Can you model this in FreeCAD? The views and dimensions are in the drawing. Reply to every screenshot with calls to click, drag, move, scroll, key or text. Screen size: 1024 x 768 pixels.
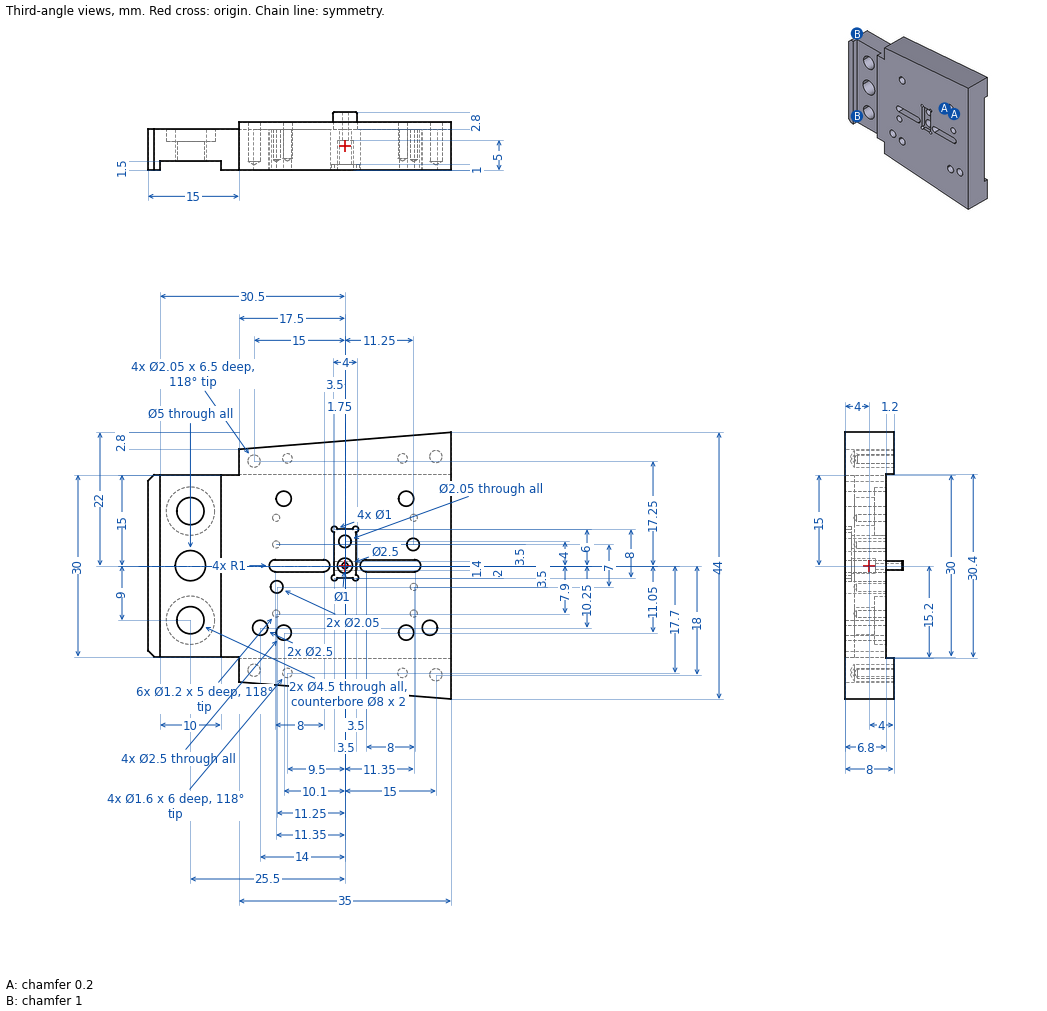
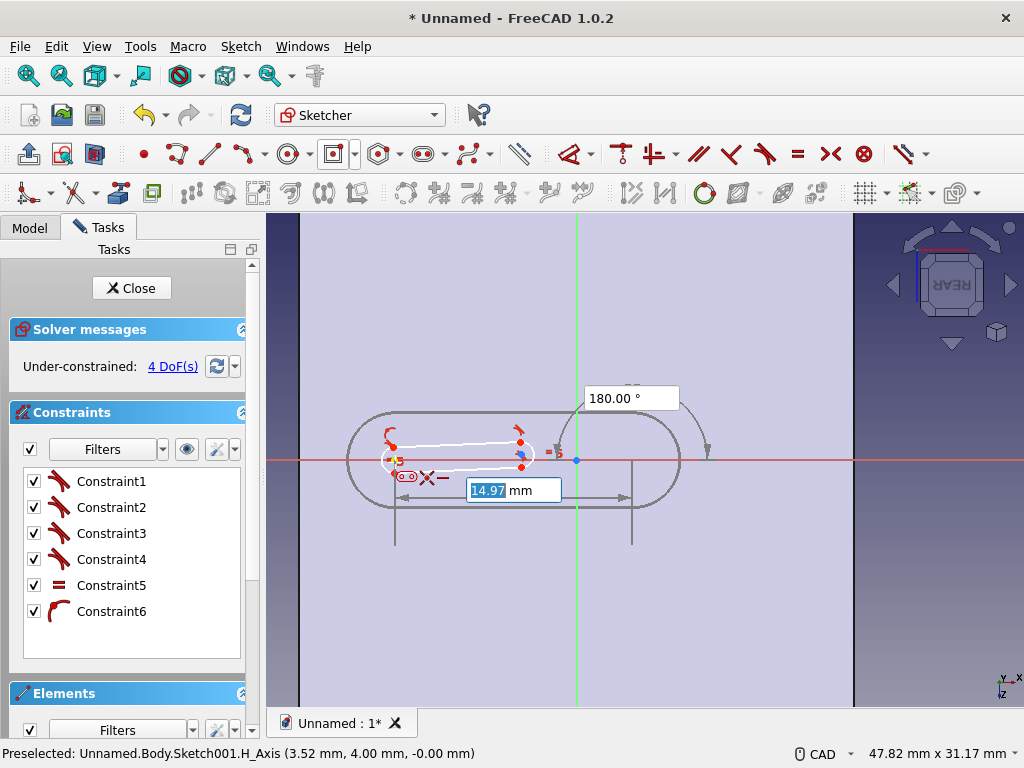
click(759, 451)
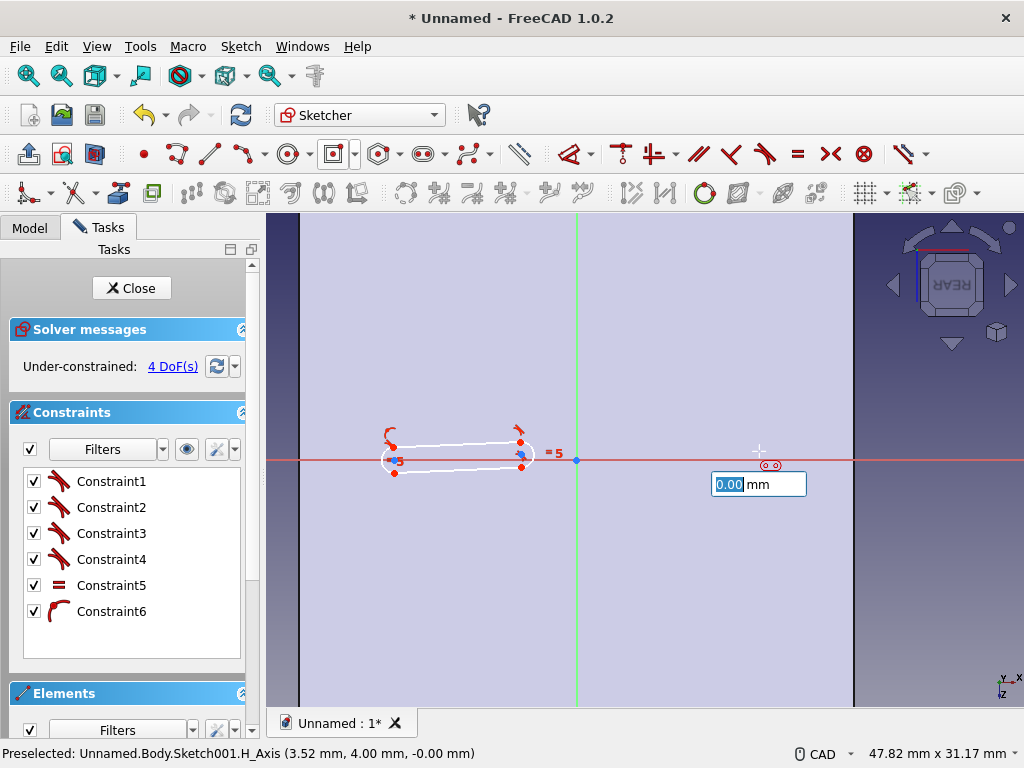
click(695, 444)
key(Escape)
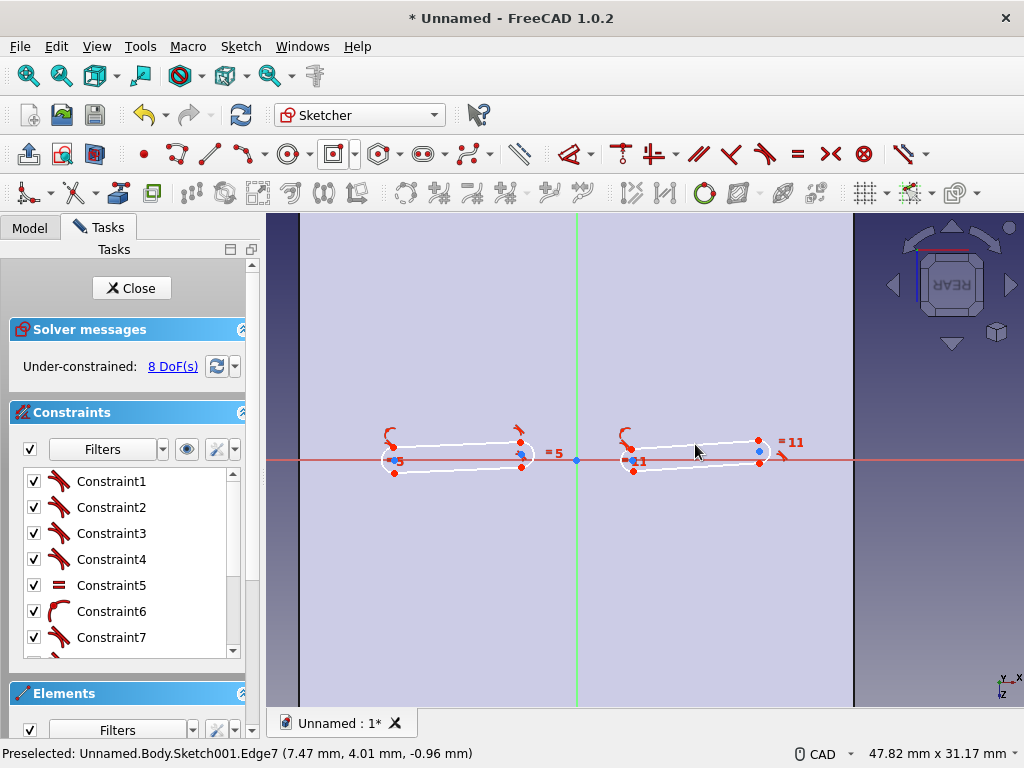
click(432, 446)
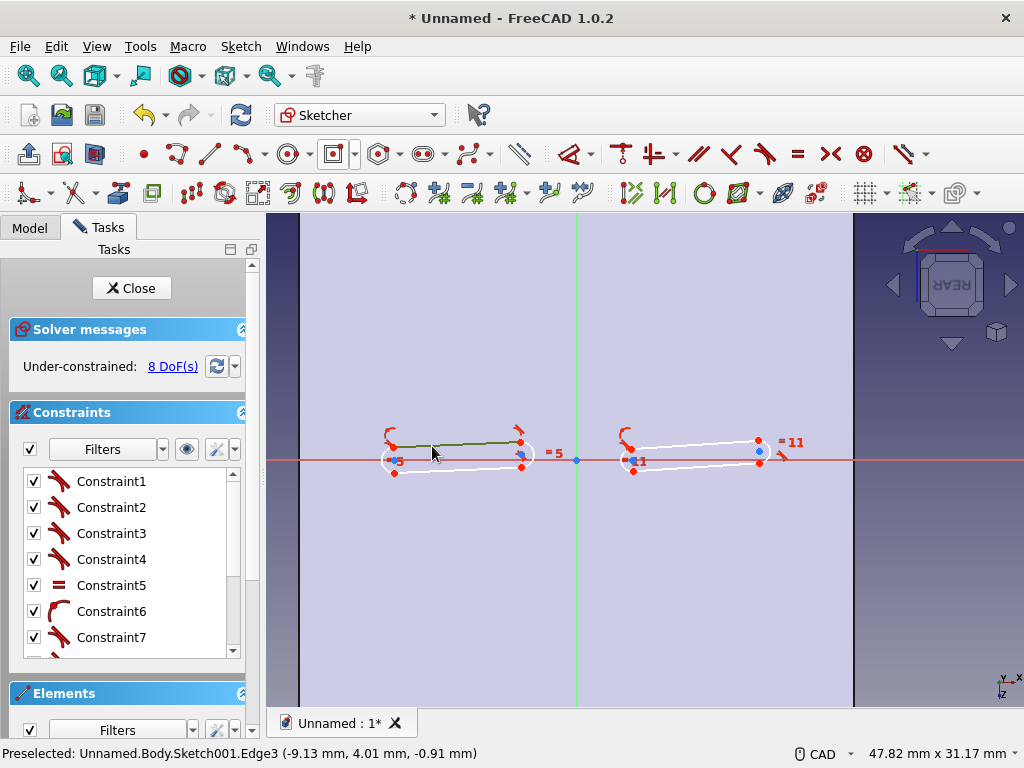
click(676, 154)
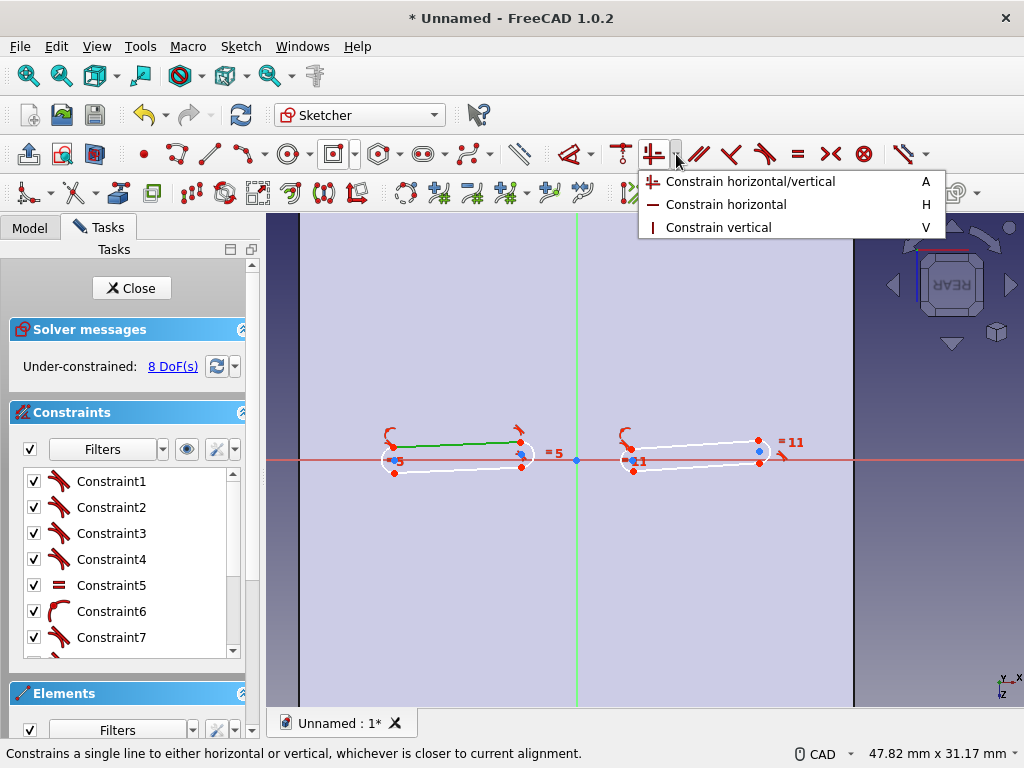
click(792, 204)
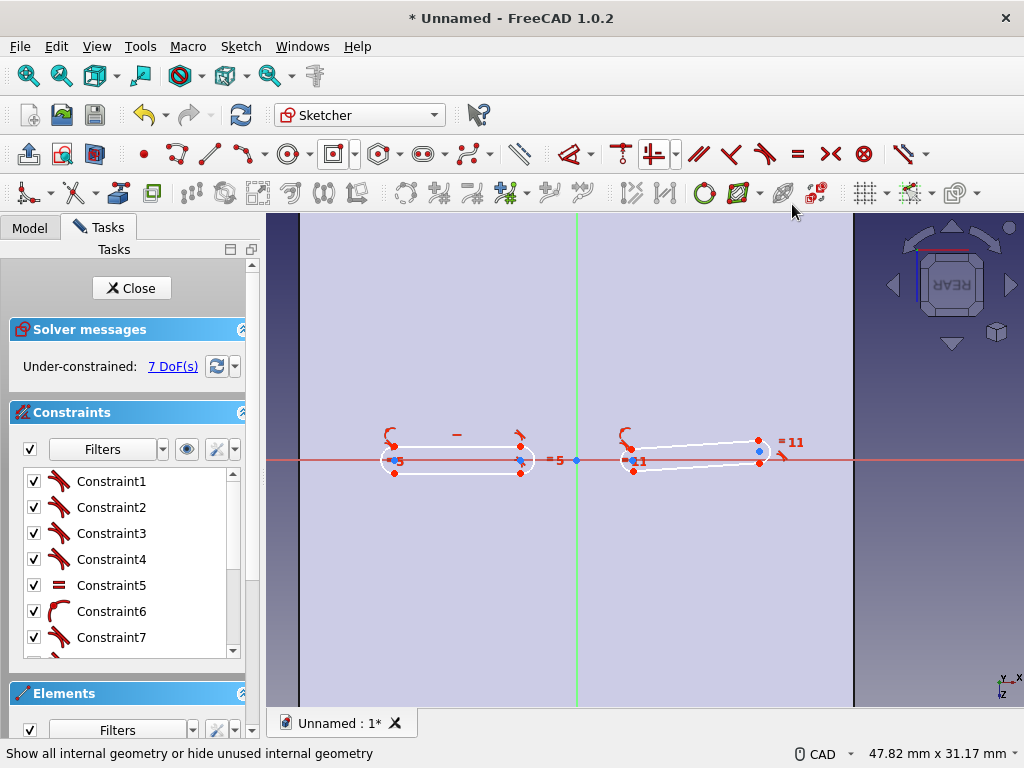
click(670, 447)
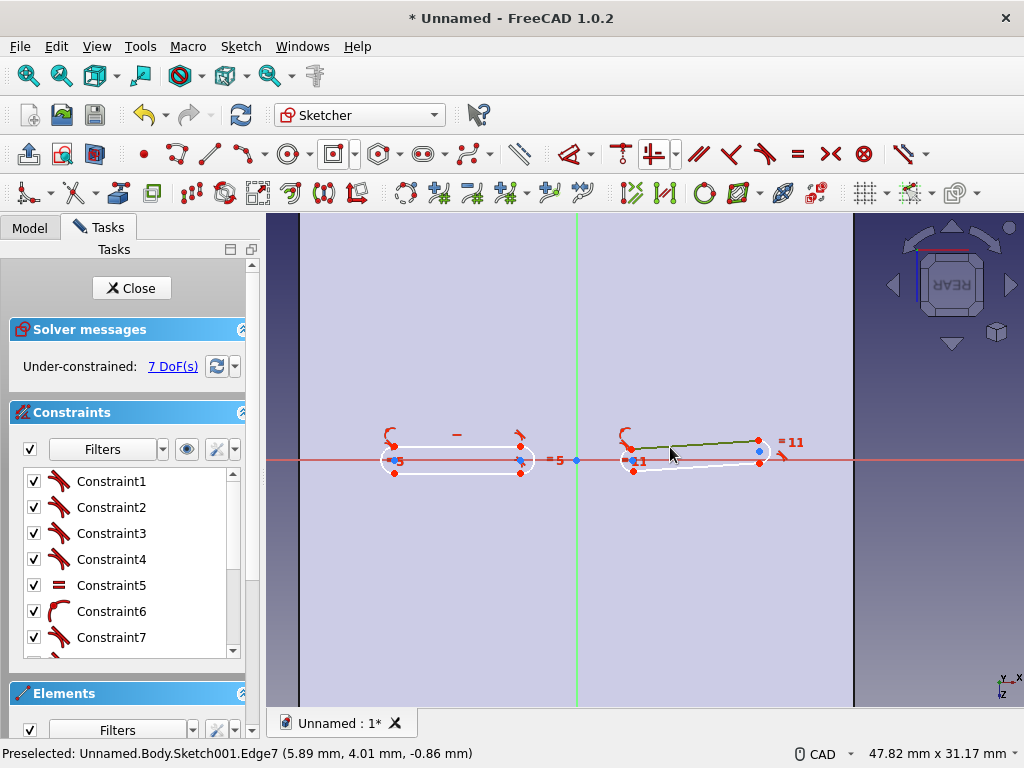
click(676, 154)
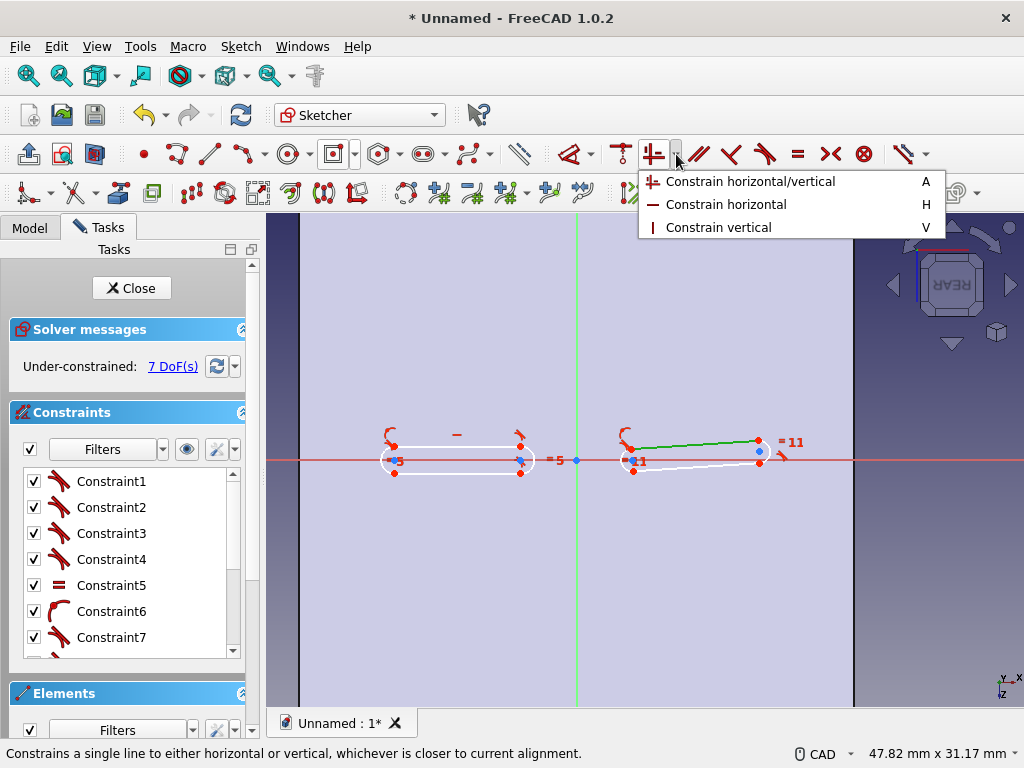
click(792, 204)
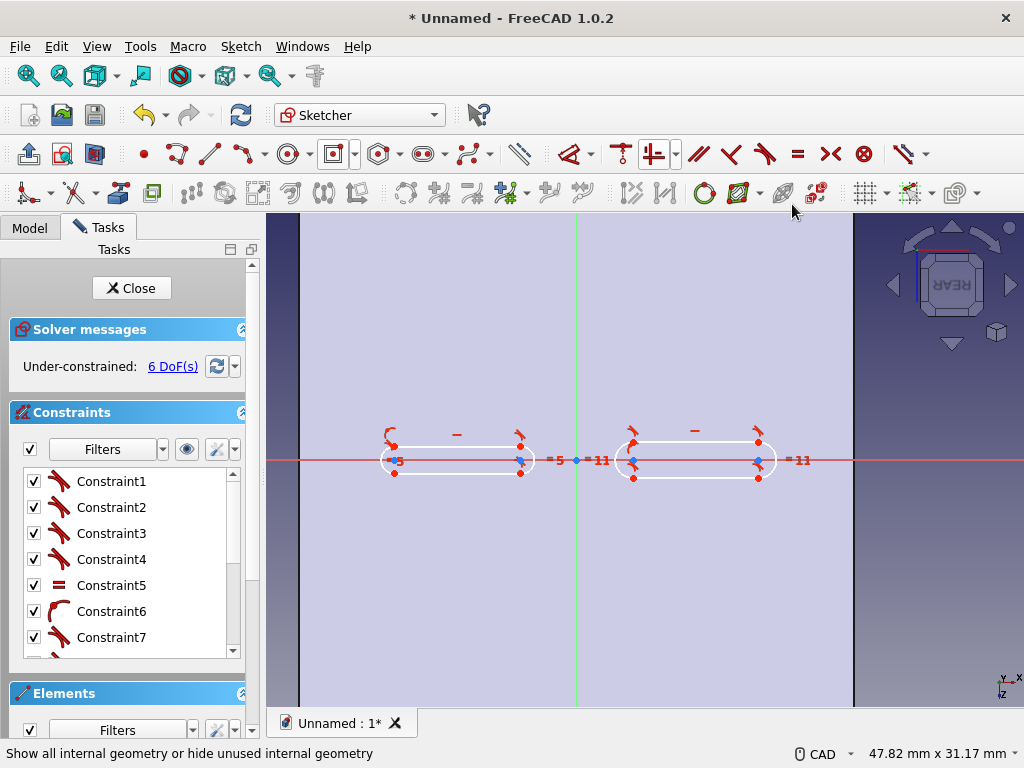
click(381, 460)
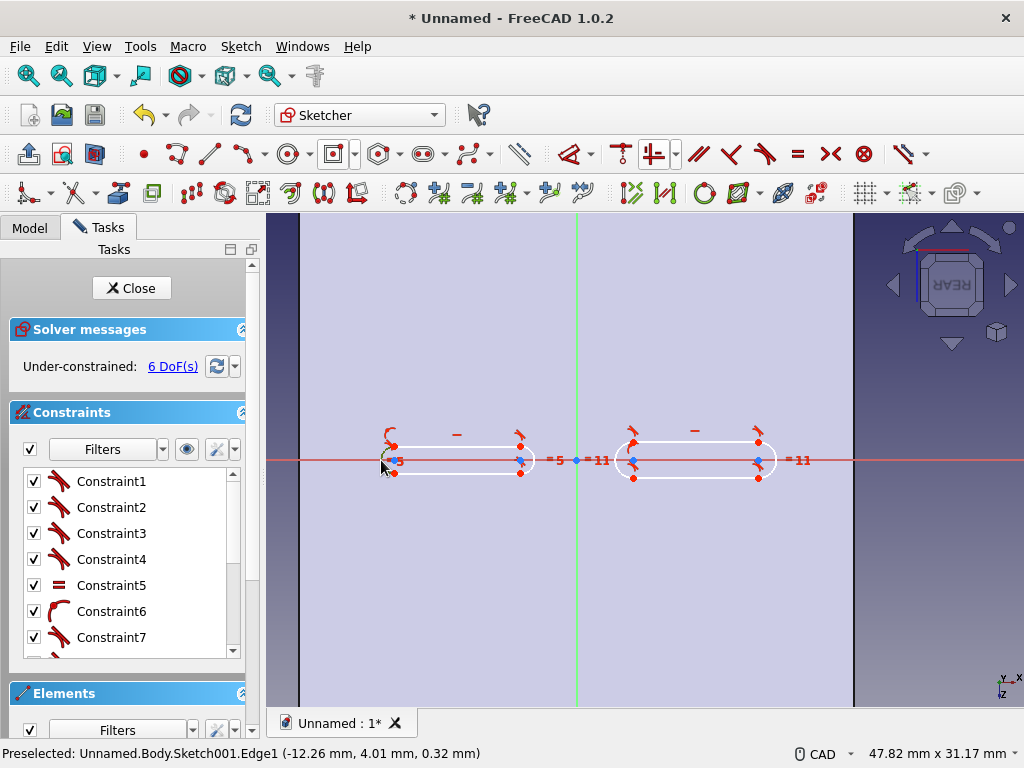
scroll(619, 450, up, 2)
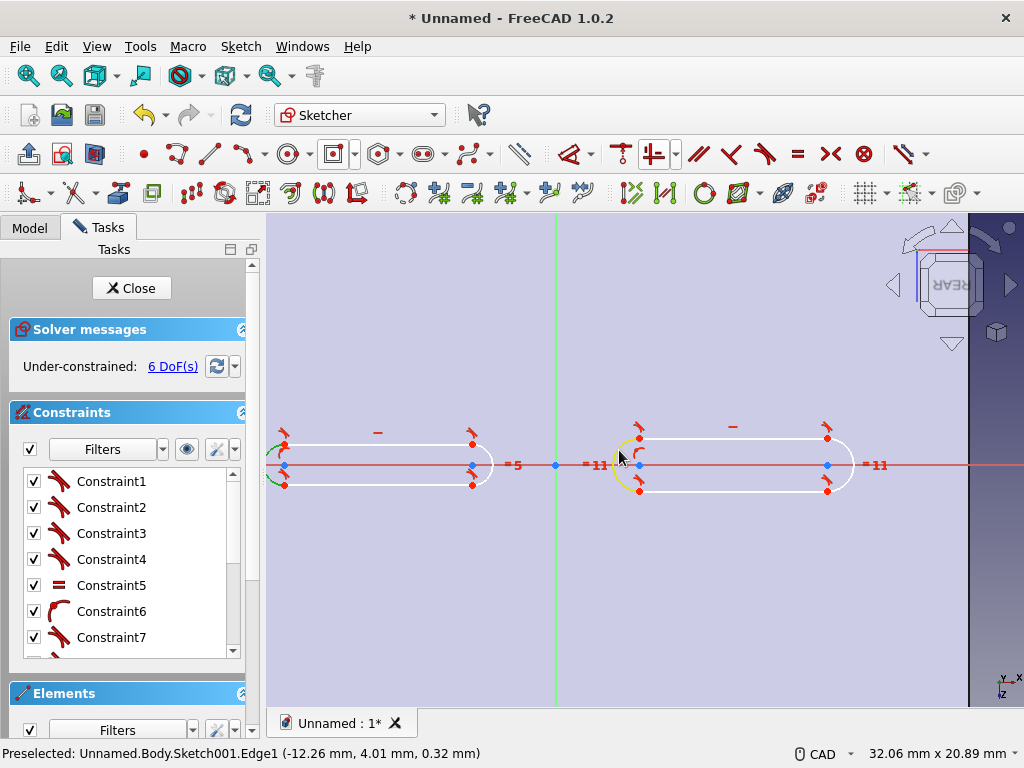
click(618, 449)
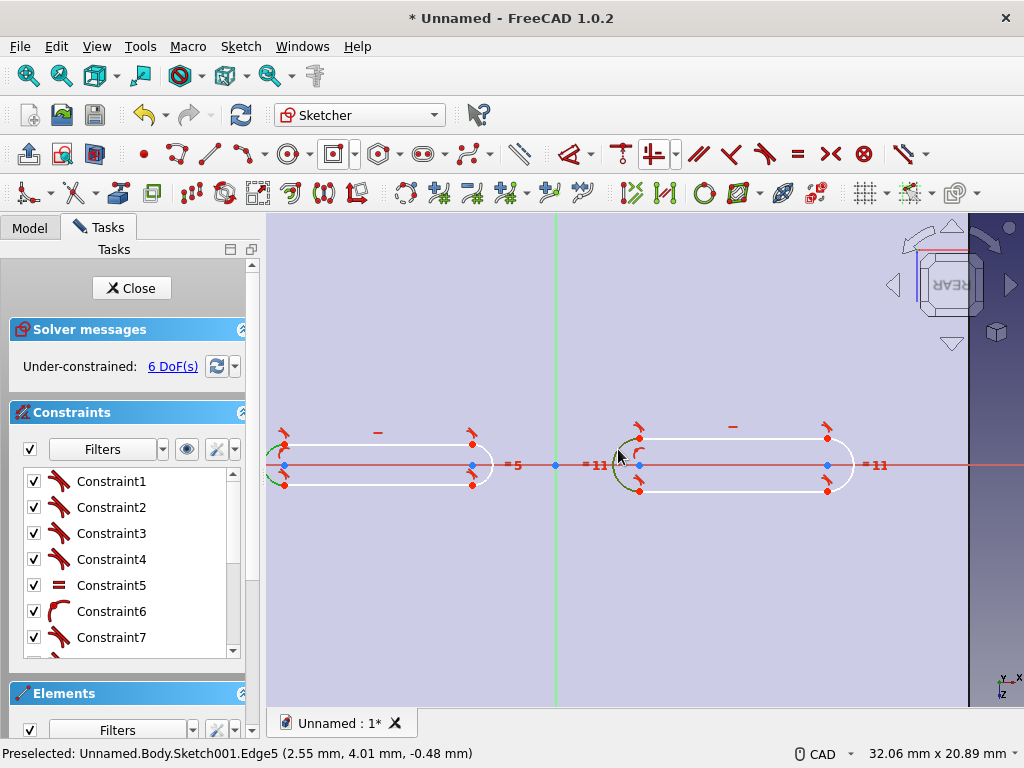
click(798, 154)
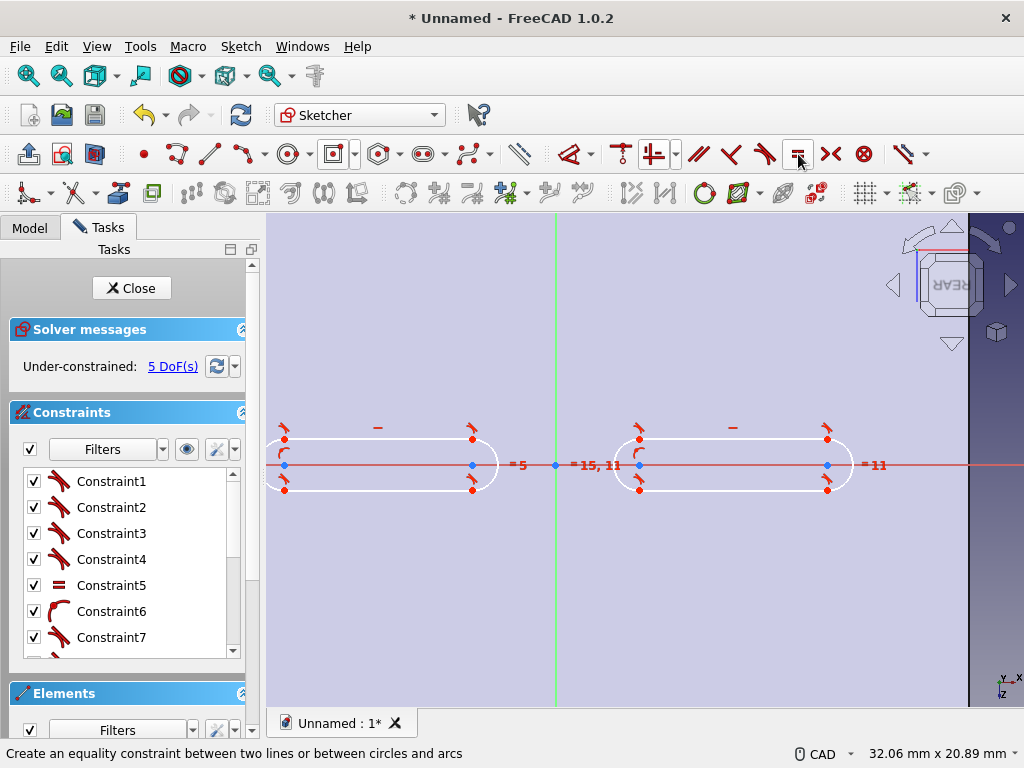
scroll(619, 450, down, 2)